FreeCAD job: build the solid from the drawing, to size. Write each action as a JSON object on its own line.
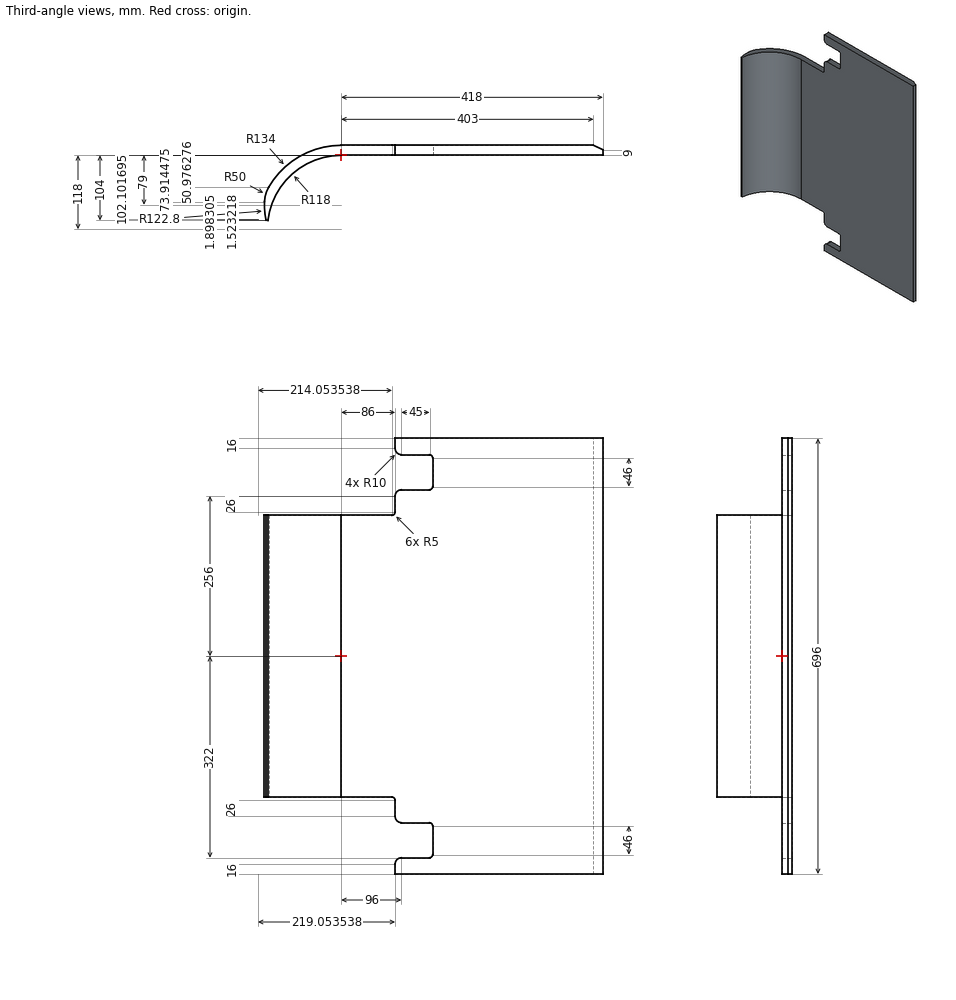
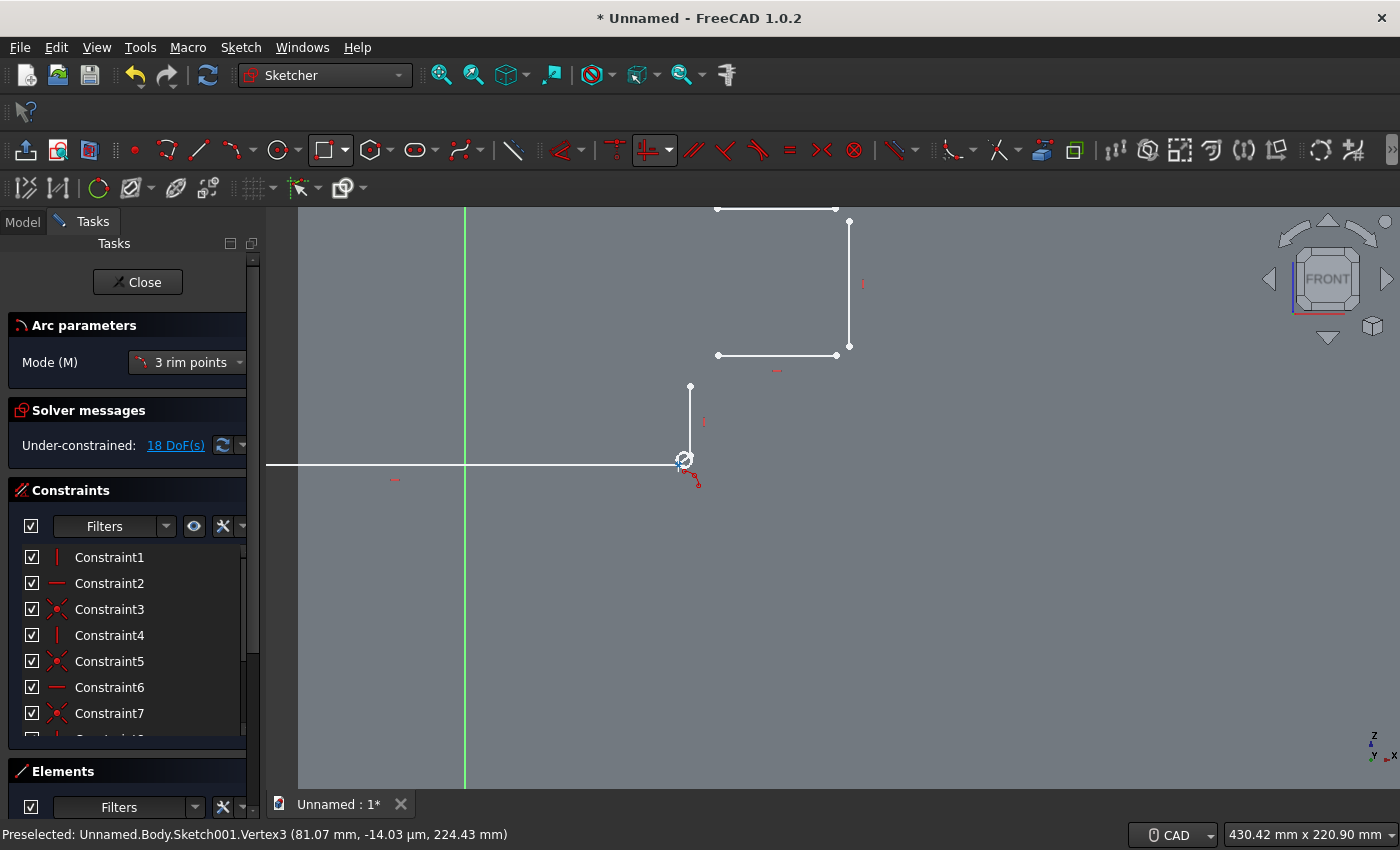
{"action": "scroll", "coordinate": [688, 459], "scroll_direction": "up", "scroll_amount": 8}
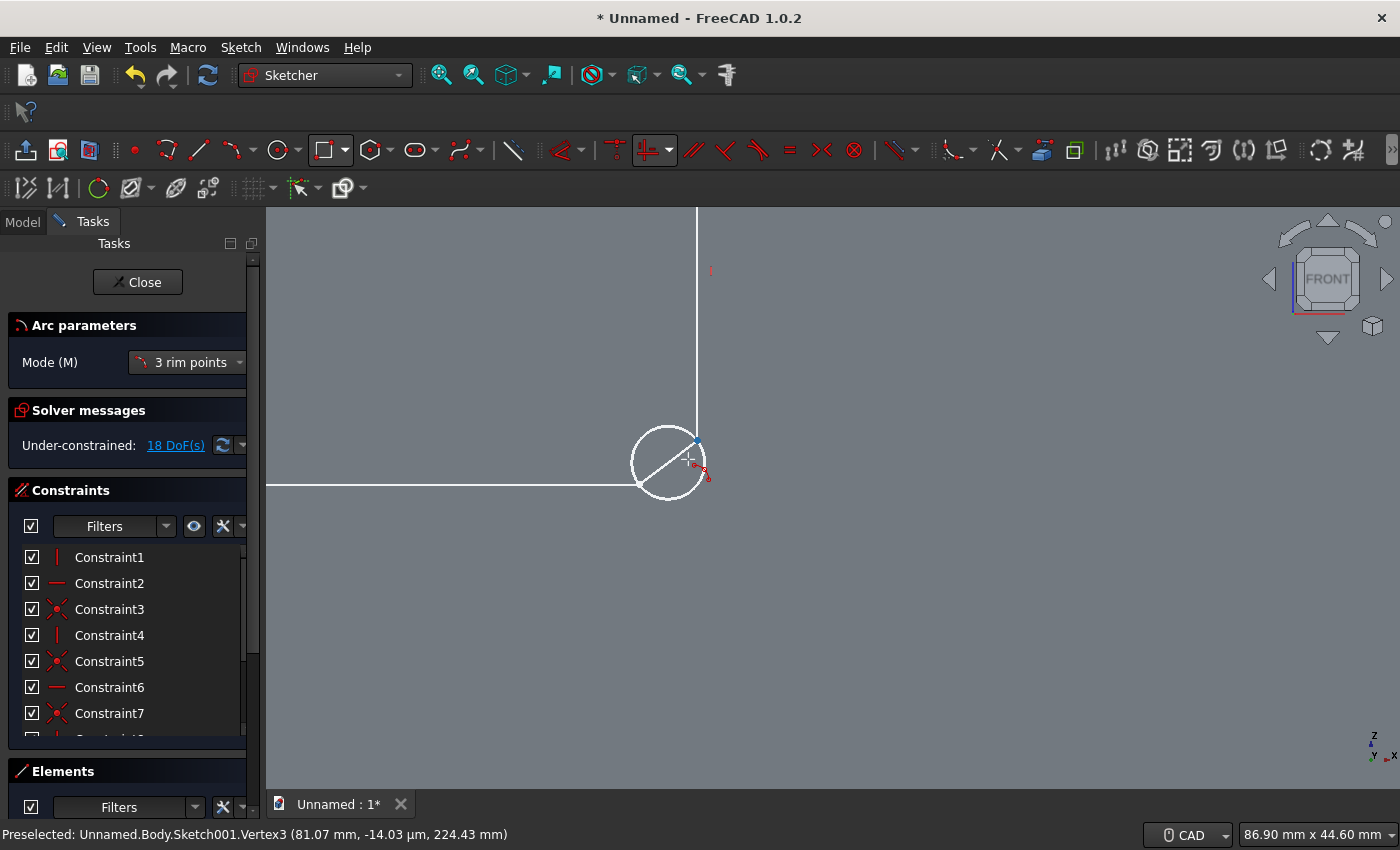
{"action": "left_click", "coordinate": [684, 458]}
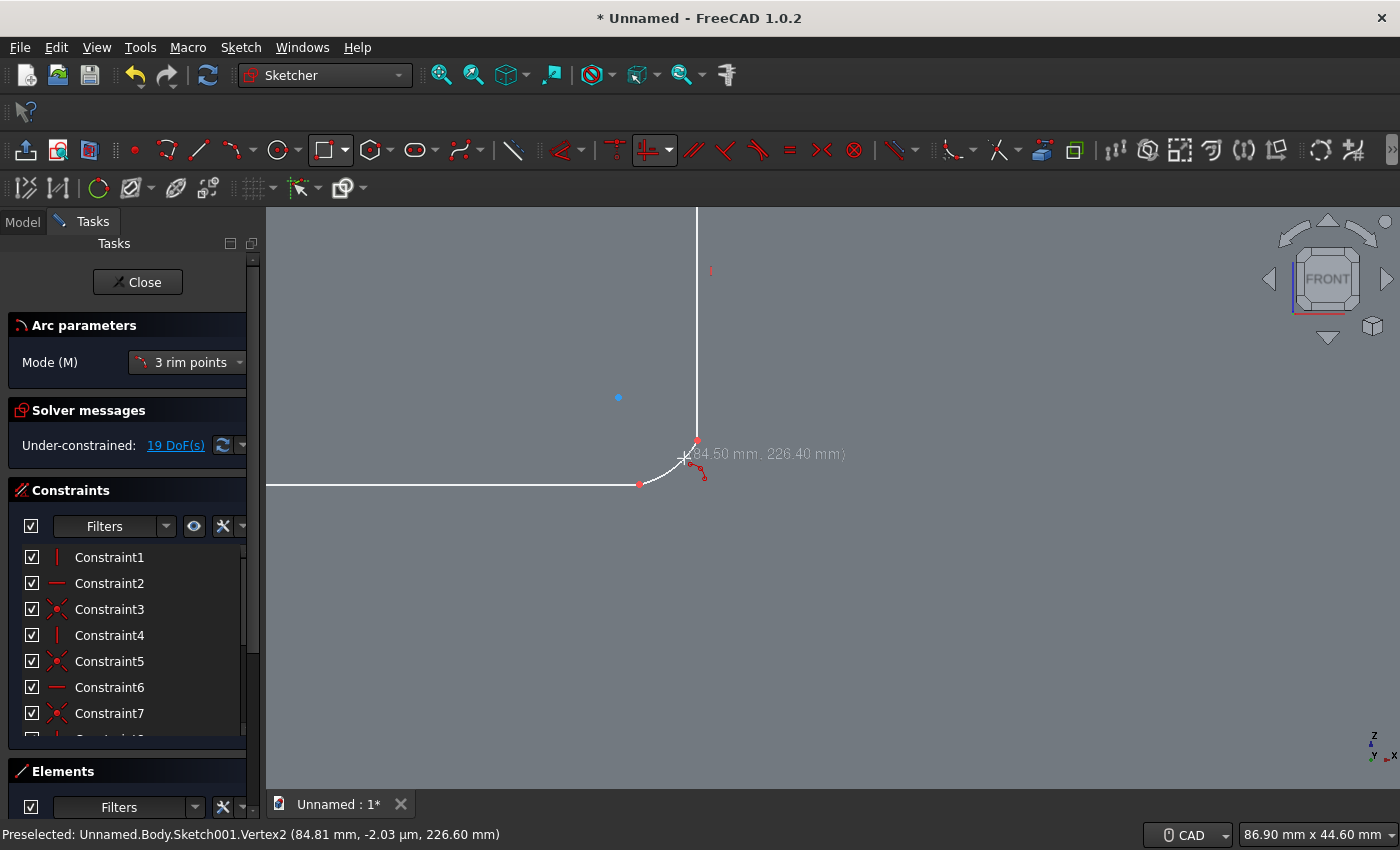
{"action": "scroll", "coordinate": [822, 345], "scroll_direction": "down", "scroll_amount": 15}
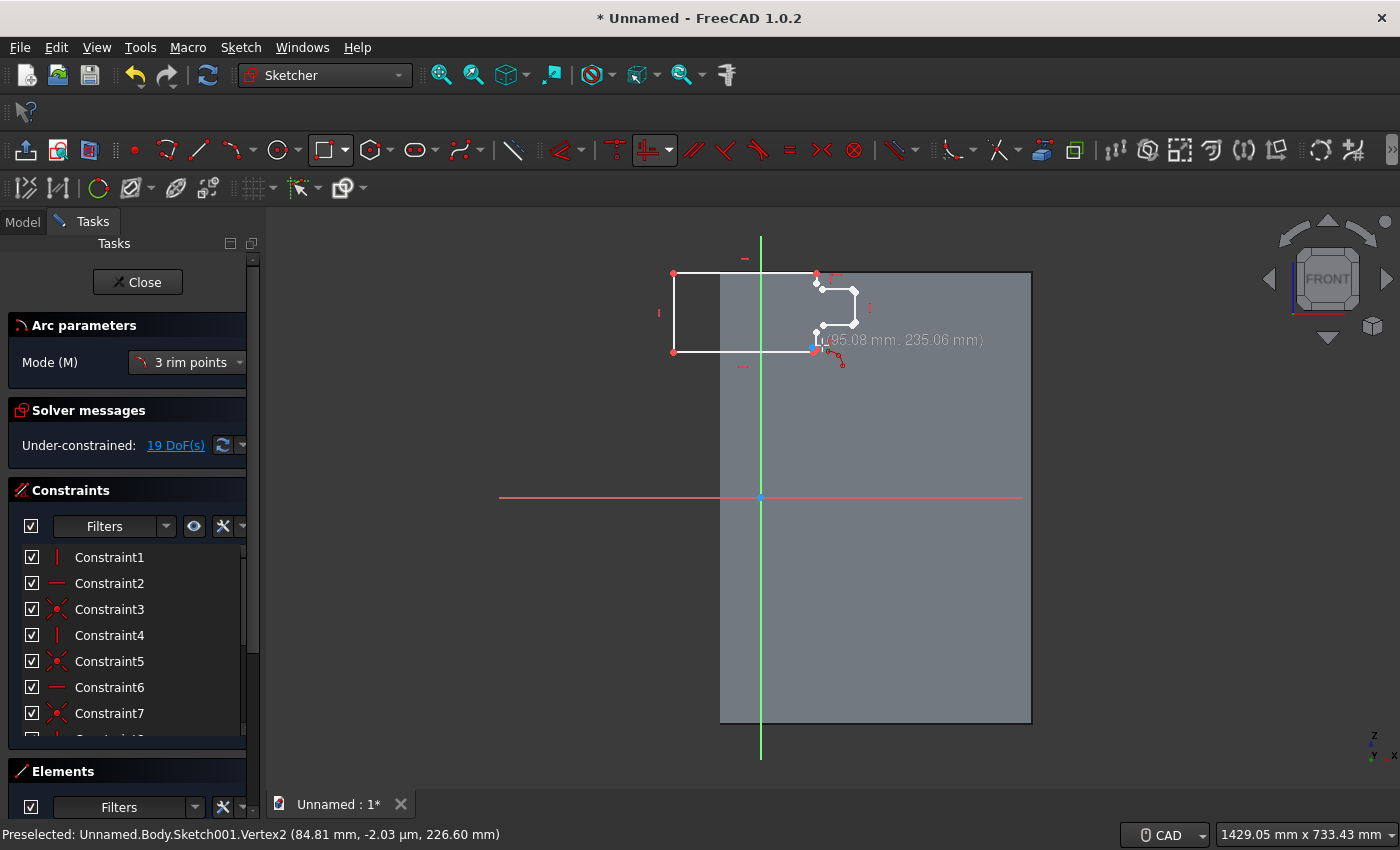
{"action": "scroll", "coordinate": [817, 282], "scroll_direction": "up", "scroll_amount": 6}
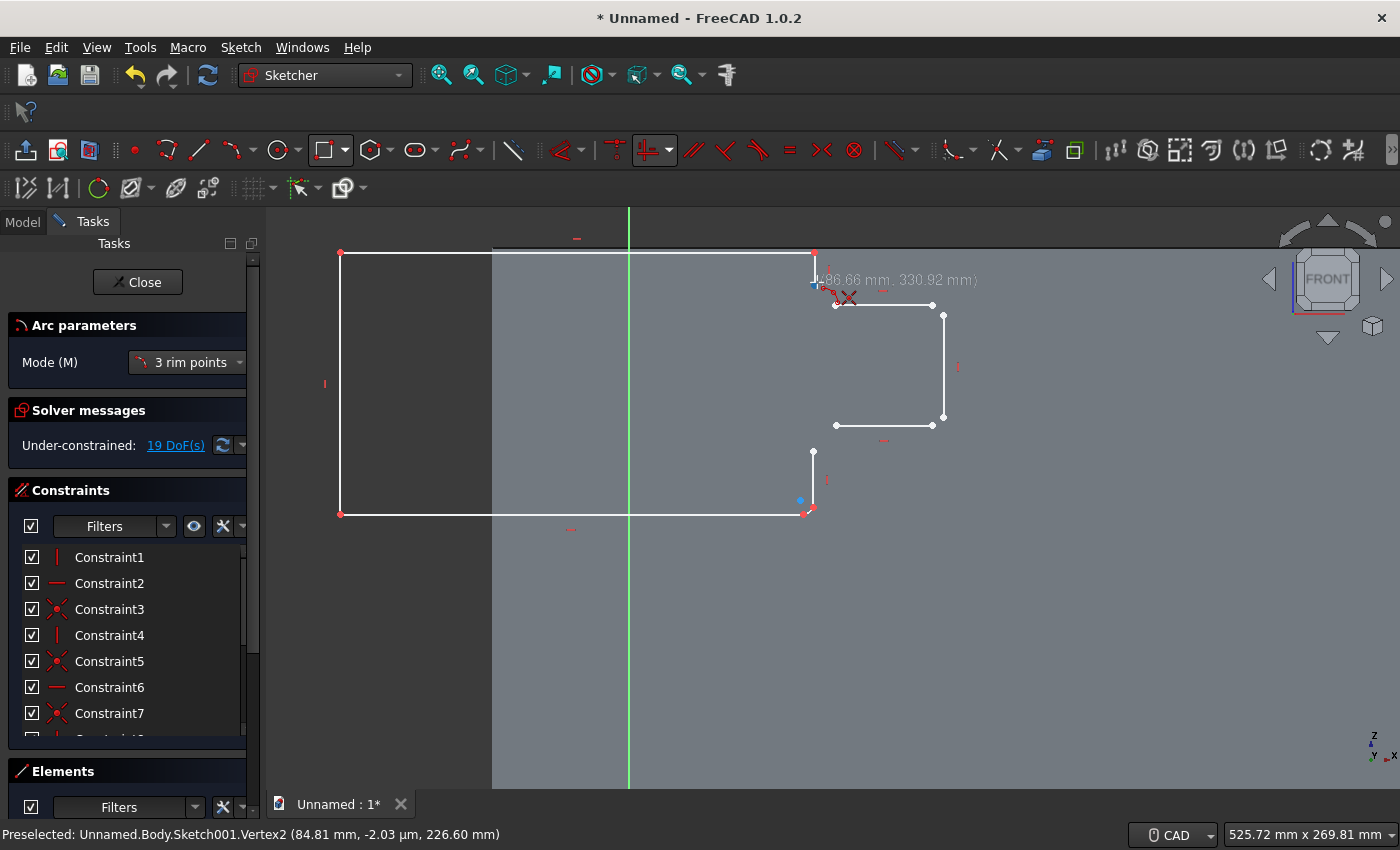
{"action": "left_click", "coordinate": [815, 285]}
{"action": "left_click", "coordinate": [836, 305]}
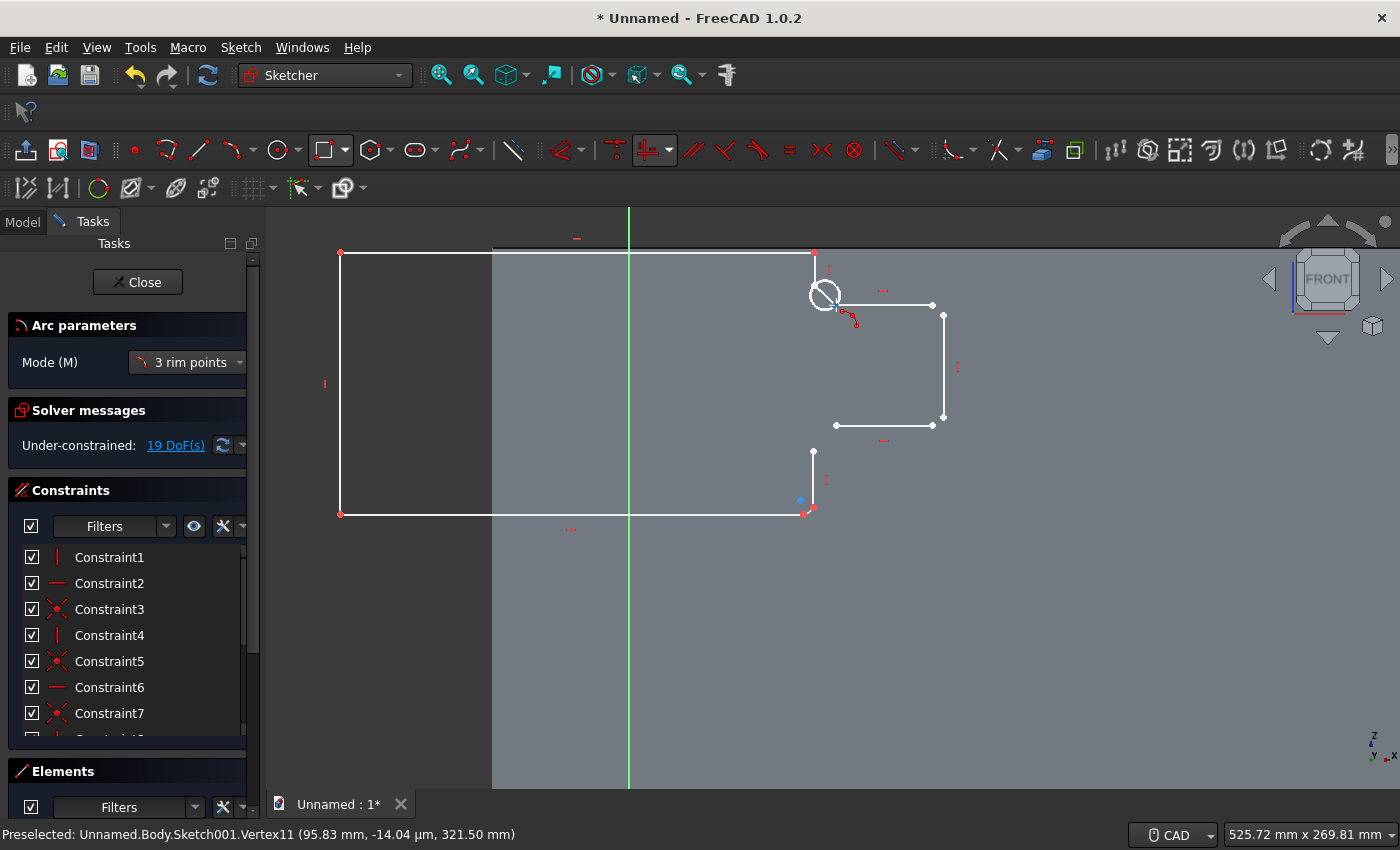
{"action": "scroll", "coordinate": [821, 298], "scroll_direction": "up", "scroll_amount": 5}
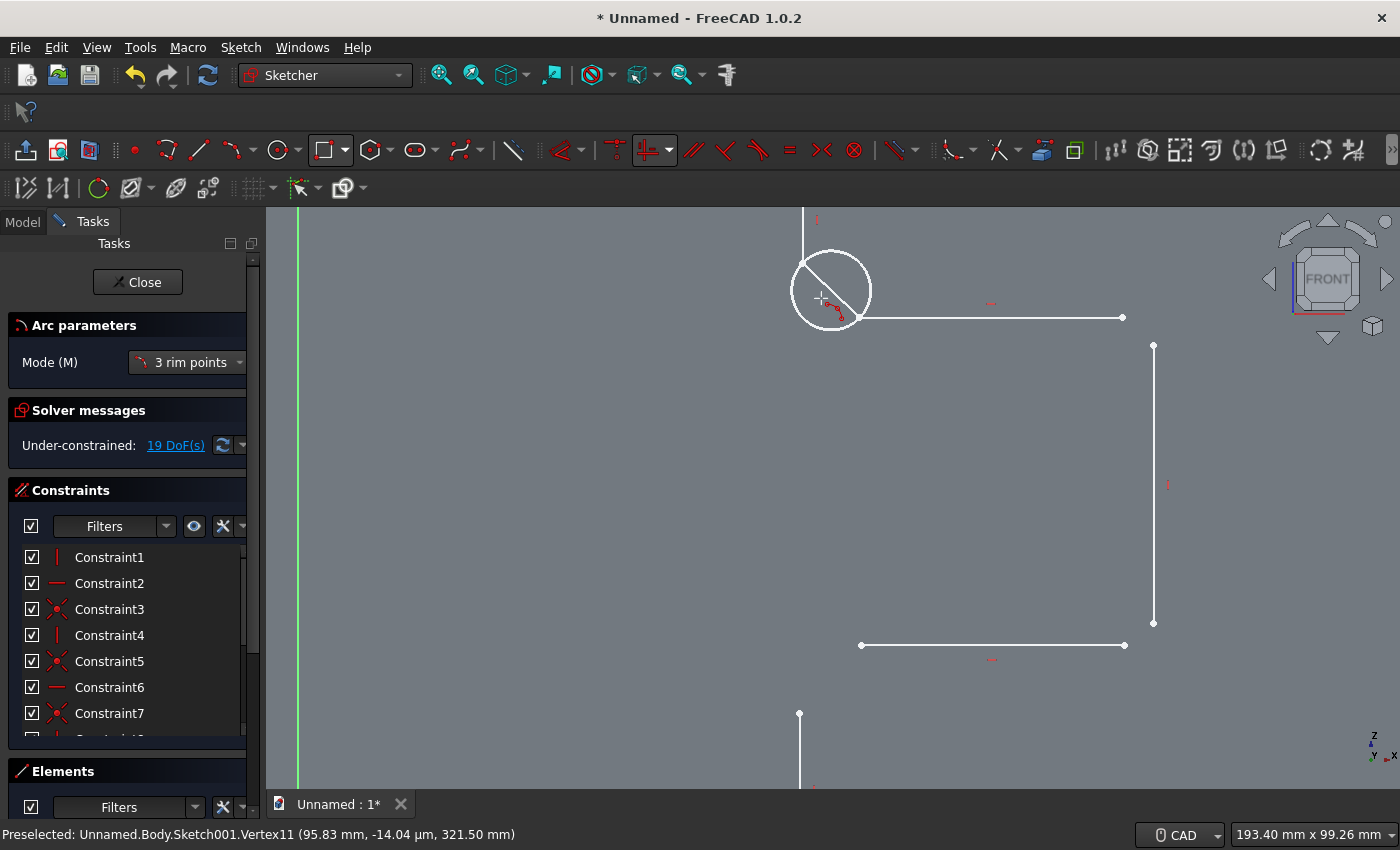
{"action": "left_click", "coordinate": [820, 298]}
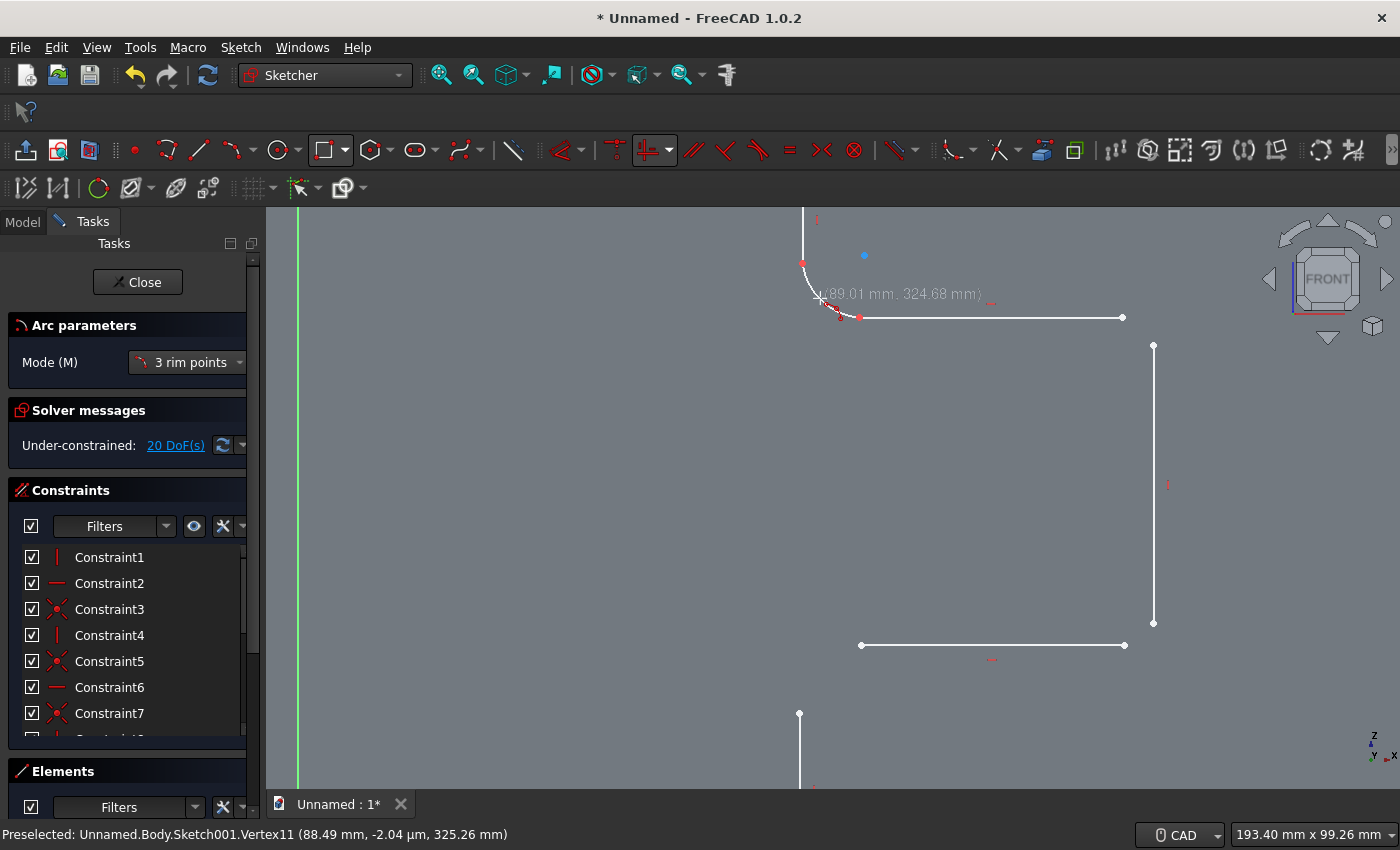
{"action": "left_click", "coordinate": [1122, 318]}
{"action": "left_click", "coordinate": [1154, 345]}